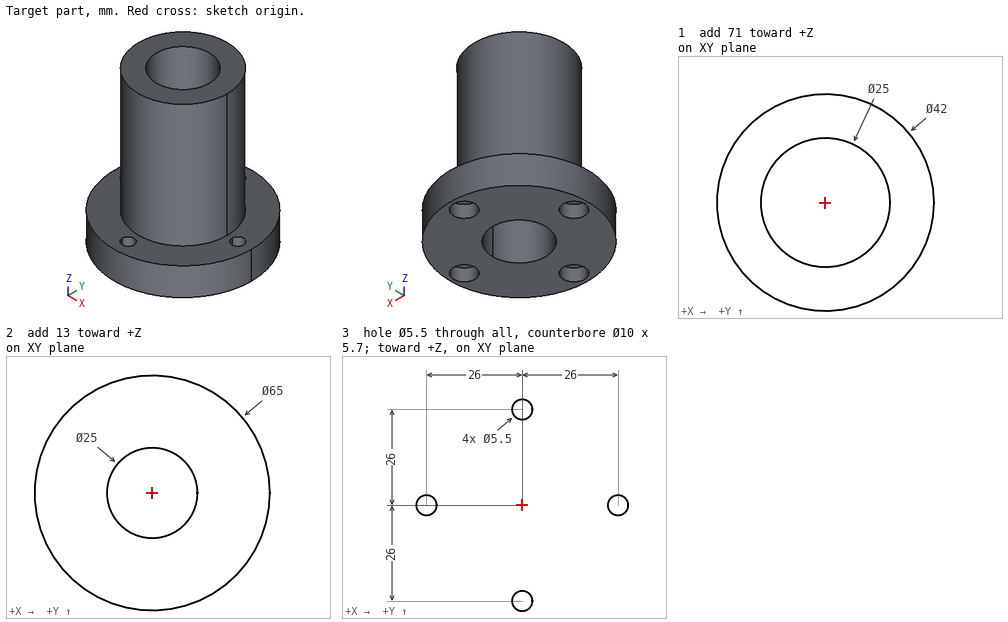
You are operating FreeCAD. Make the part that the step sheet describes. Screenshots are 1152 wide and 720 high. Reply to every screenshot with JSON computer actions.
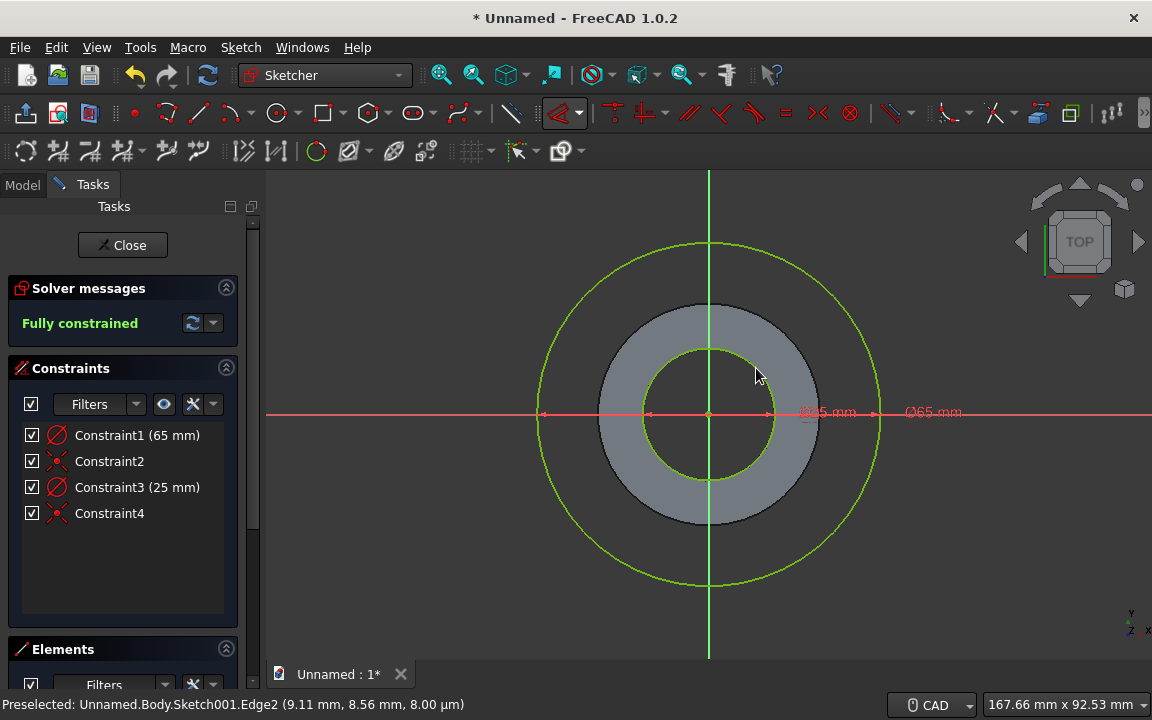
{"action": "left_click", "coordinate": [123, 245]}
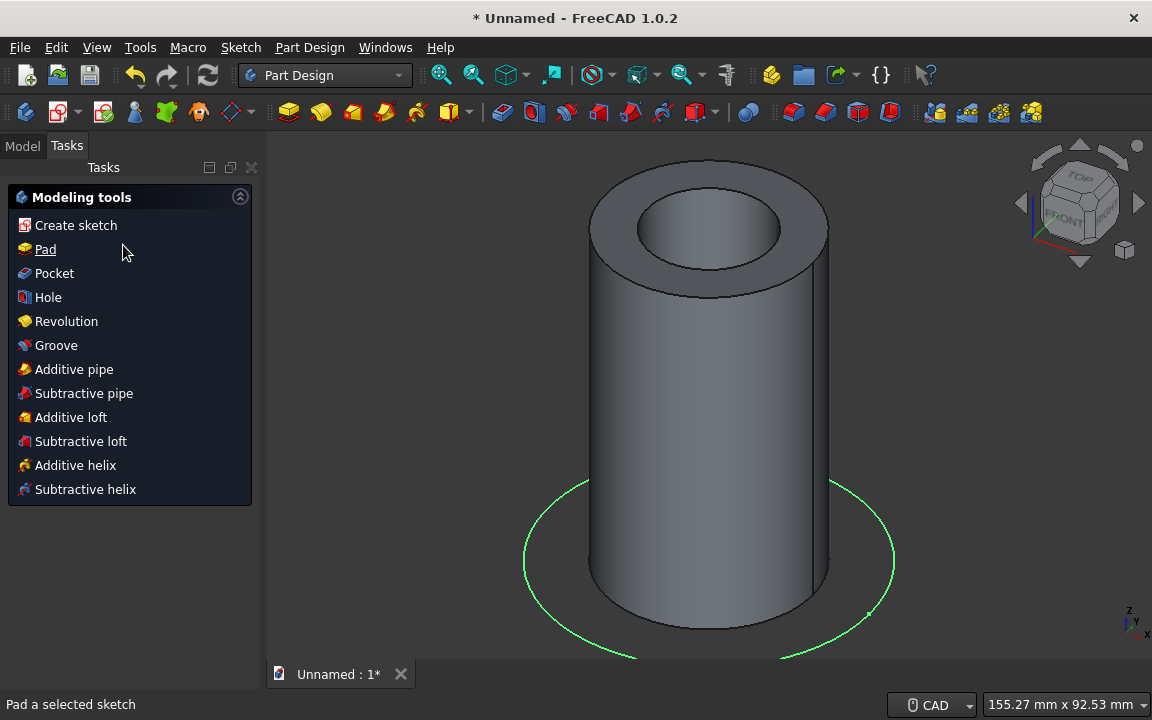
{"action": "left_click", "coordinate": [290, 112]}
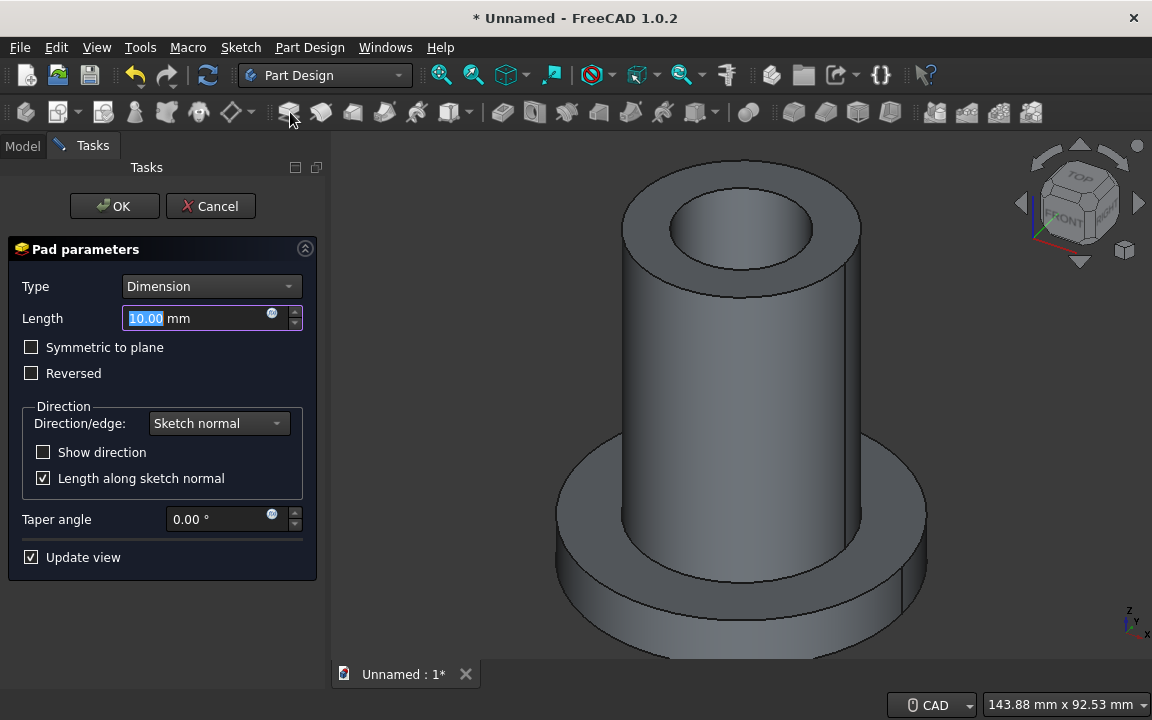
{"action": "type", "text": "13"}
{"action": "key", "text": "Tab"}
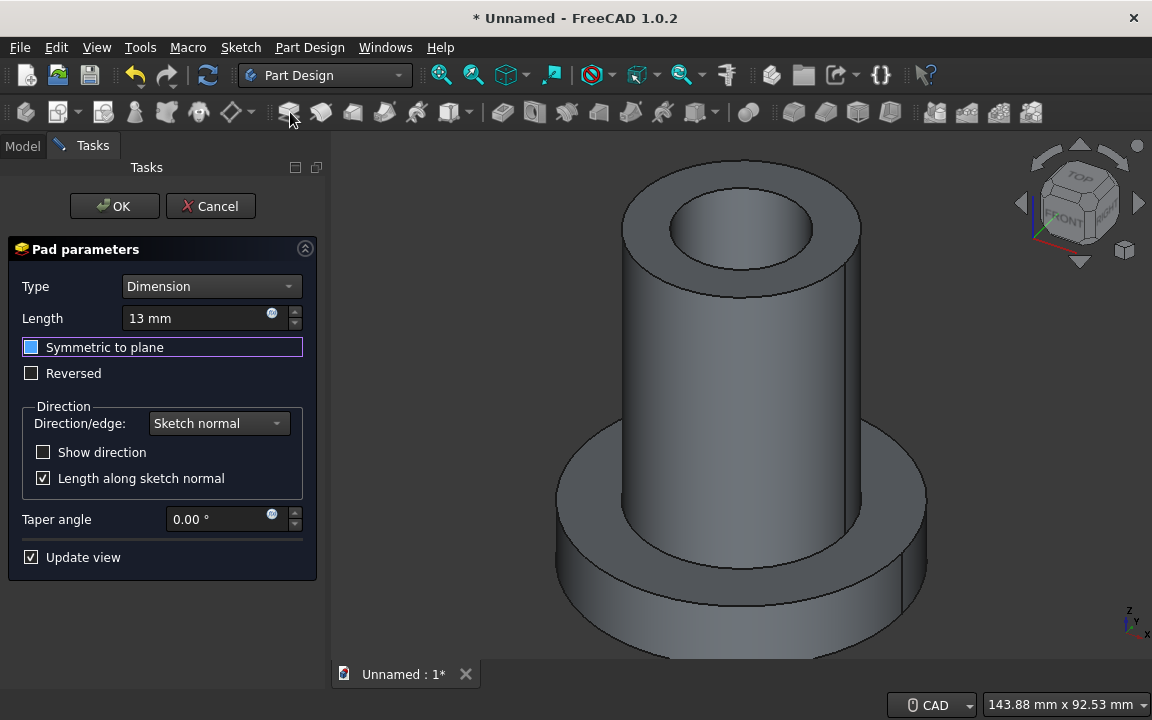
{"action": "left_click", "coordinate": [115, 206]}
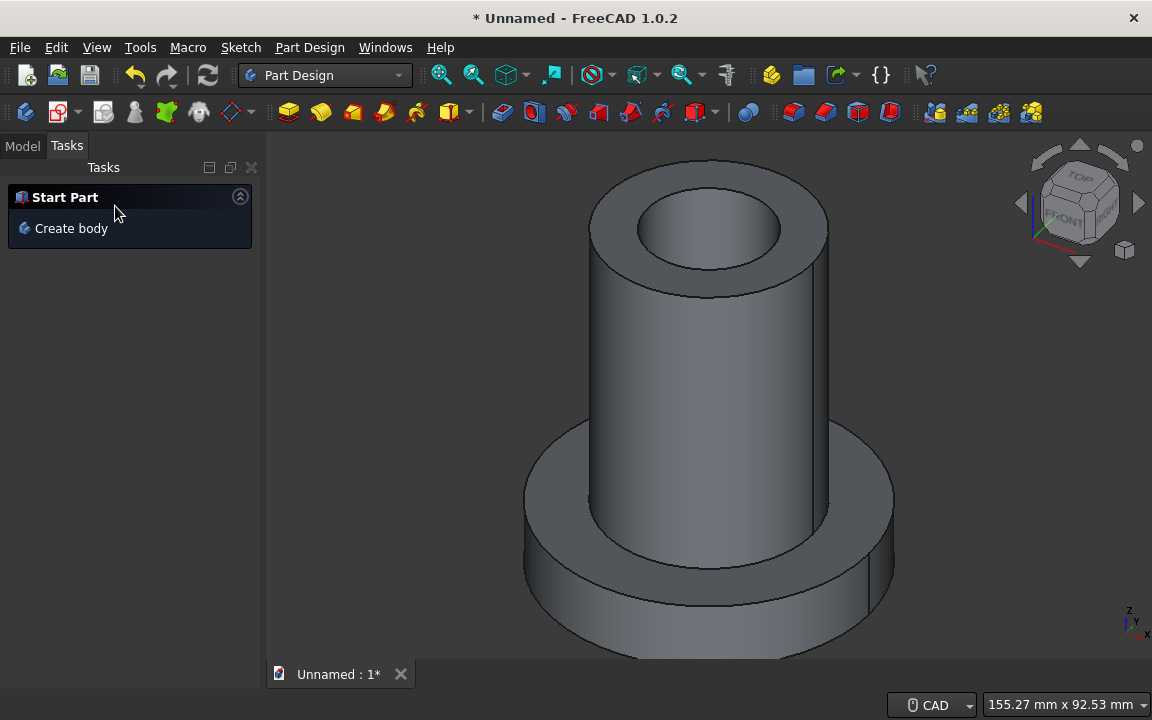
{"action": "left_click", "coordinate": [442, 76]}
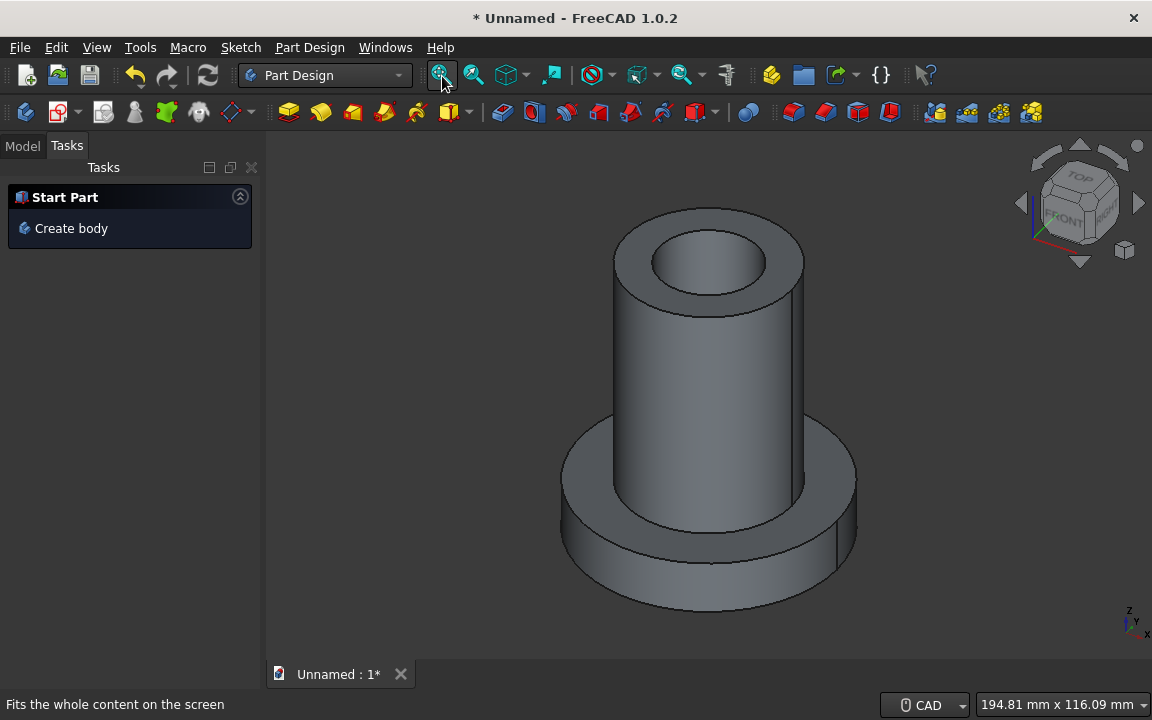
{"action": "left_click", "coordinate": [58, 112]}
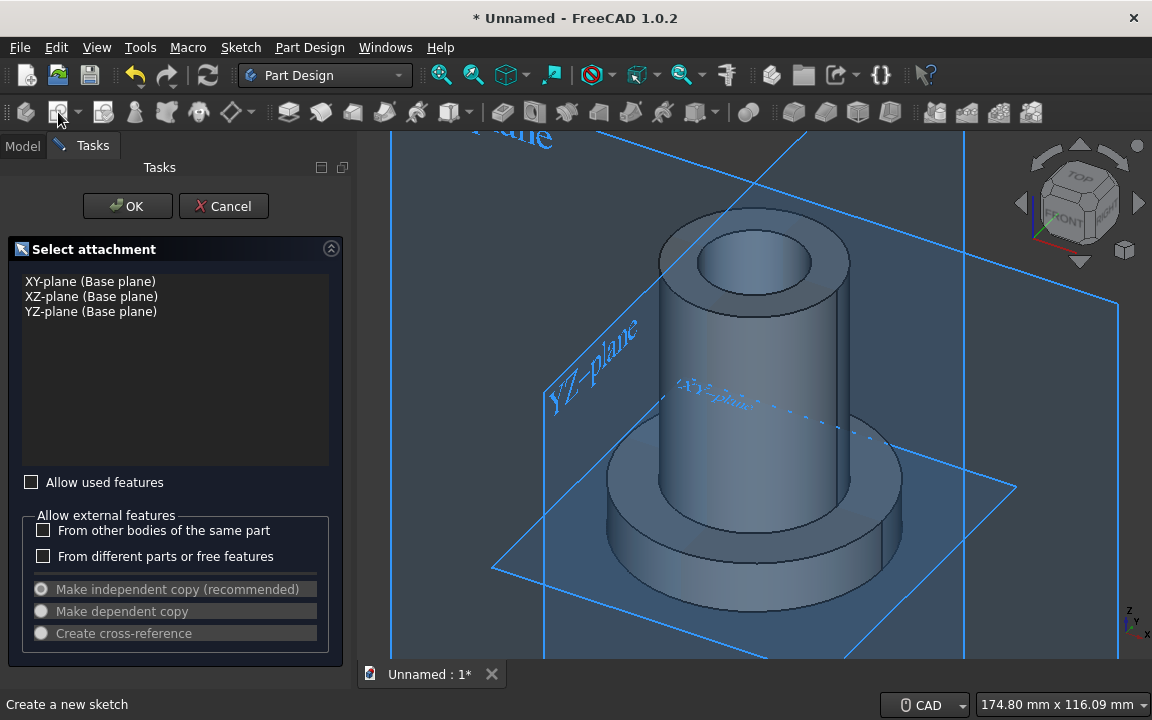
{"action": "left_click", "coordinate": [82, 282]}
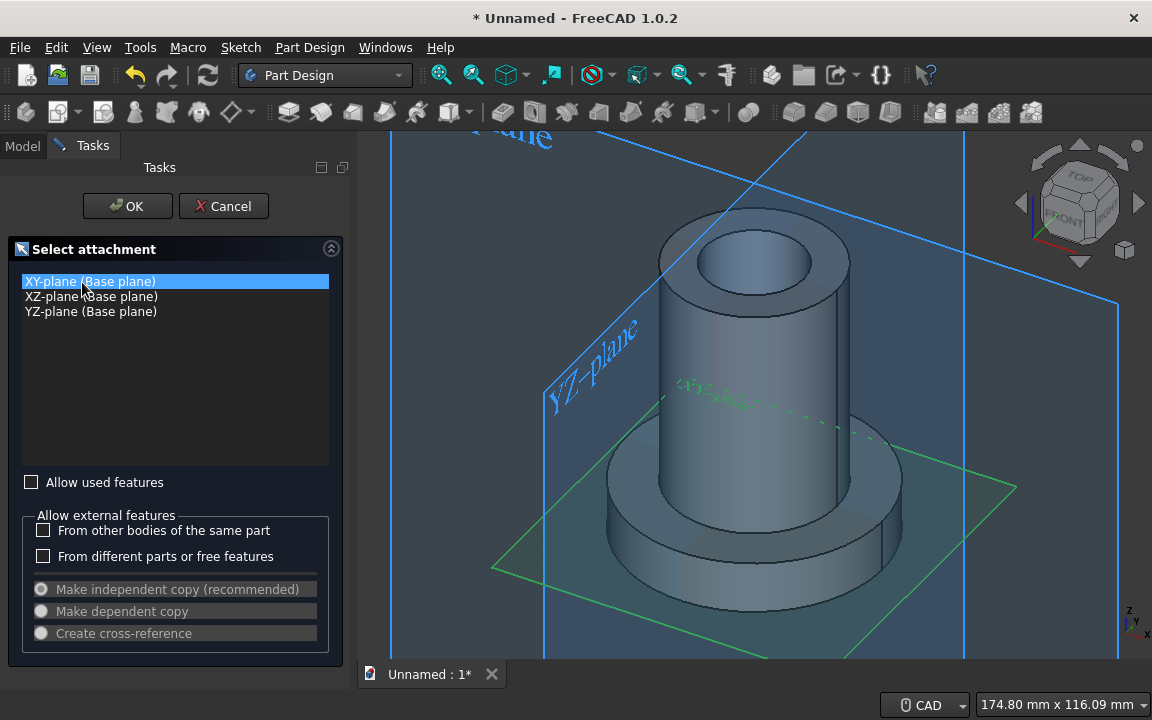
{"action": "left_click", "coordinate": [128, 206]}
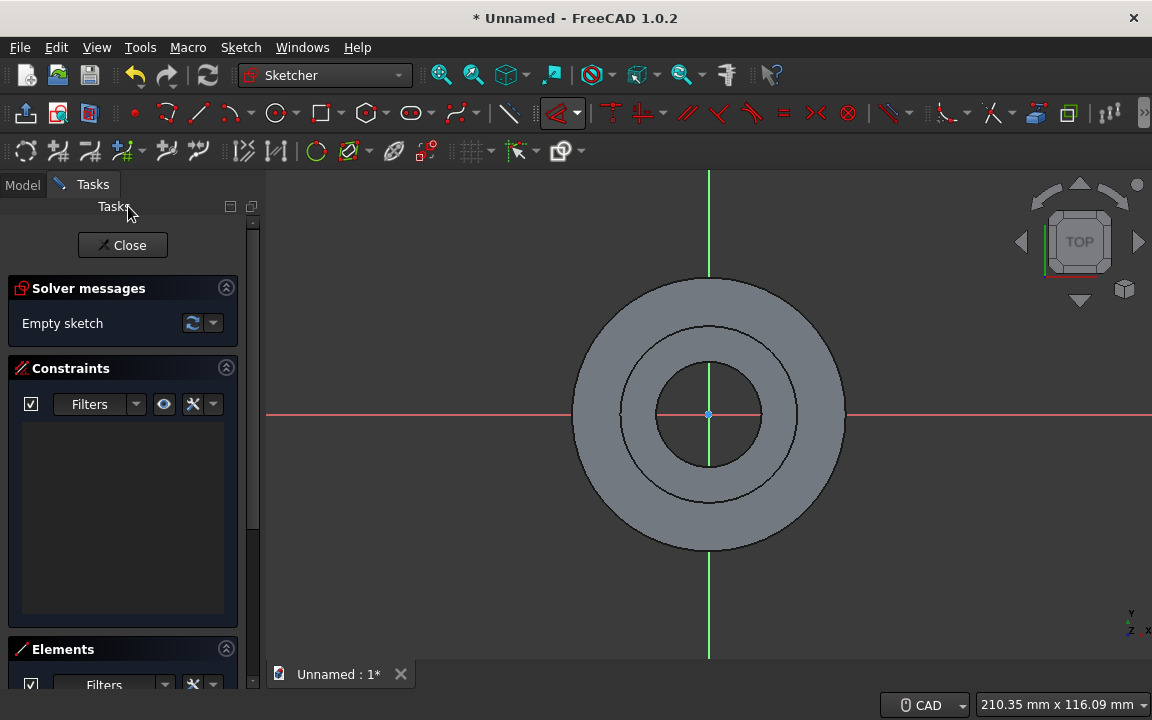
{"action": "left_click", "coordinate": [90, 114]}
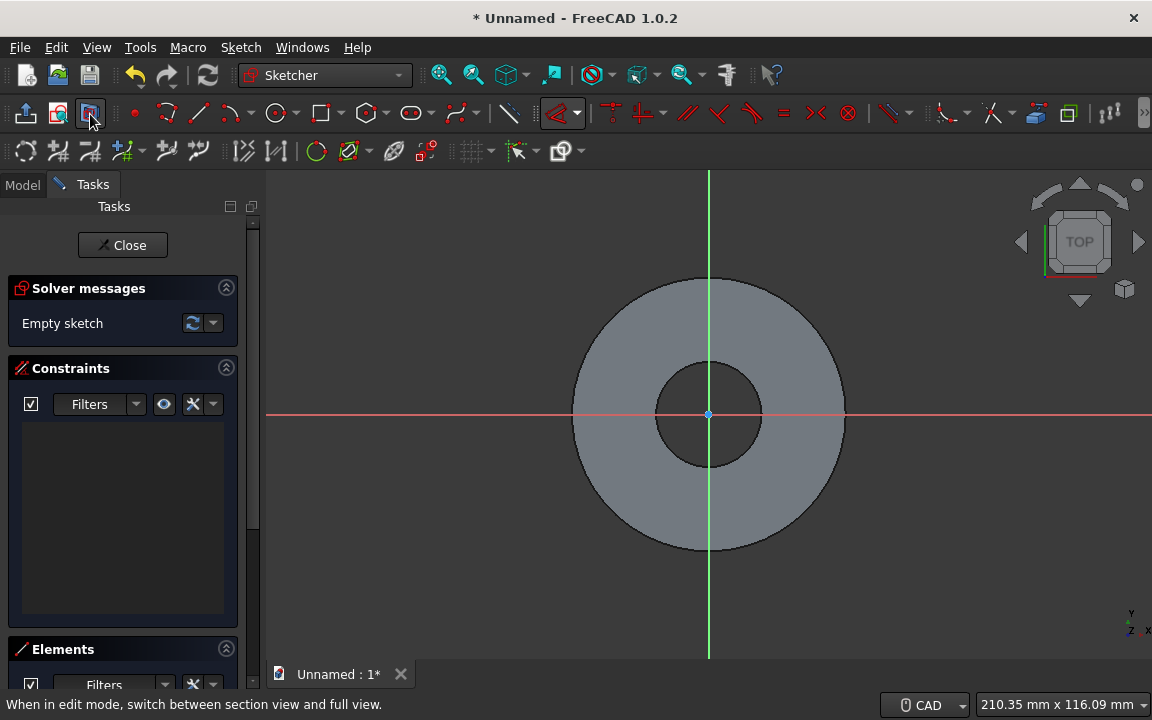
{"action": "left_click", "coordinate": [276, 114]}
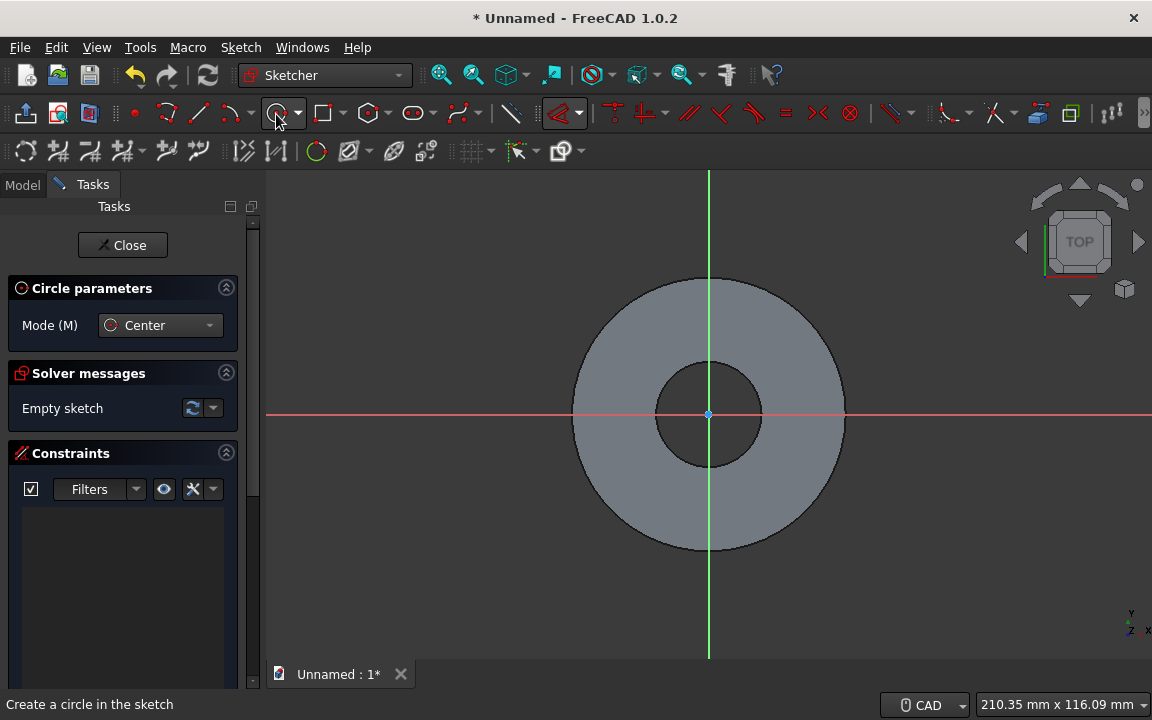
{"action": "scroll", "coordinate": [709, 305], "scroll_direction": "up", "scroll_amount": 4}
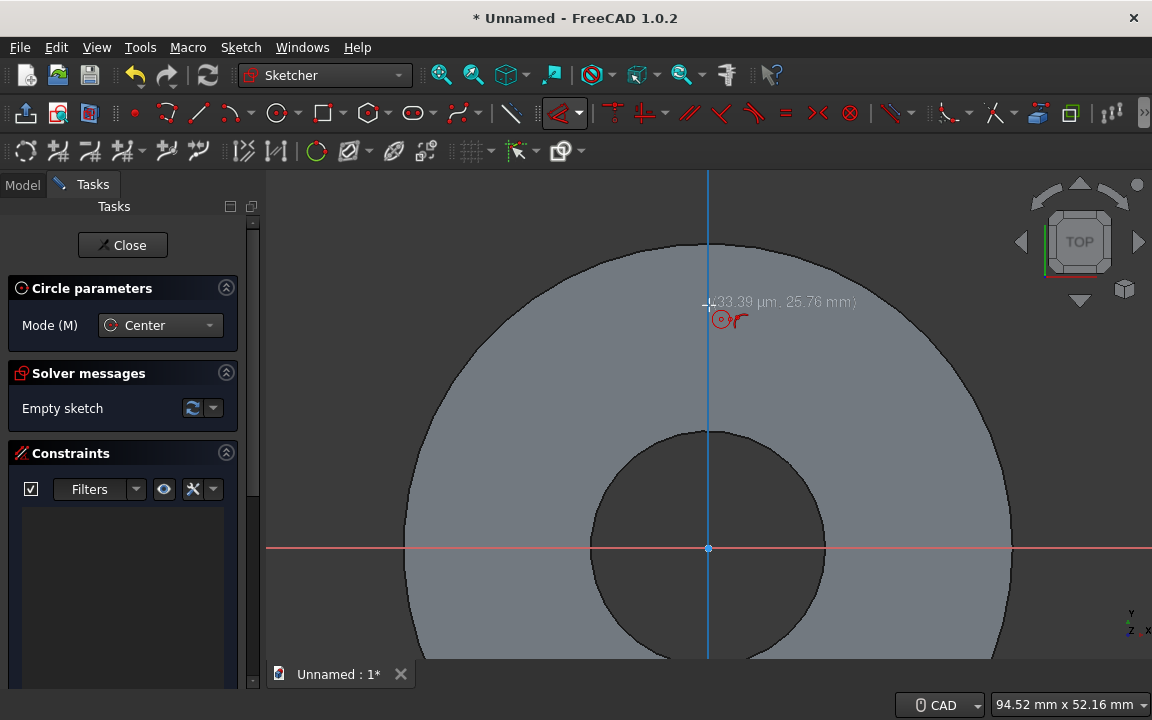
{"action": "left_click", "coordinate": [708, 305]}
{"action": "mouse_move", "coordinate": [726, 286]}